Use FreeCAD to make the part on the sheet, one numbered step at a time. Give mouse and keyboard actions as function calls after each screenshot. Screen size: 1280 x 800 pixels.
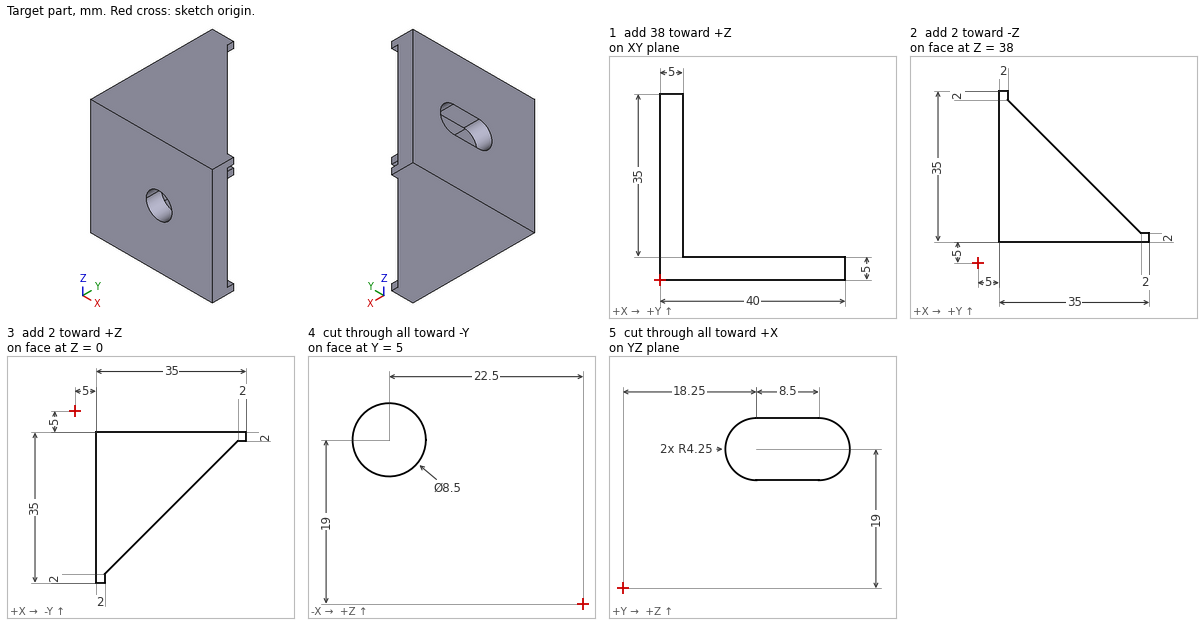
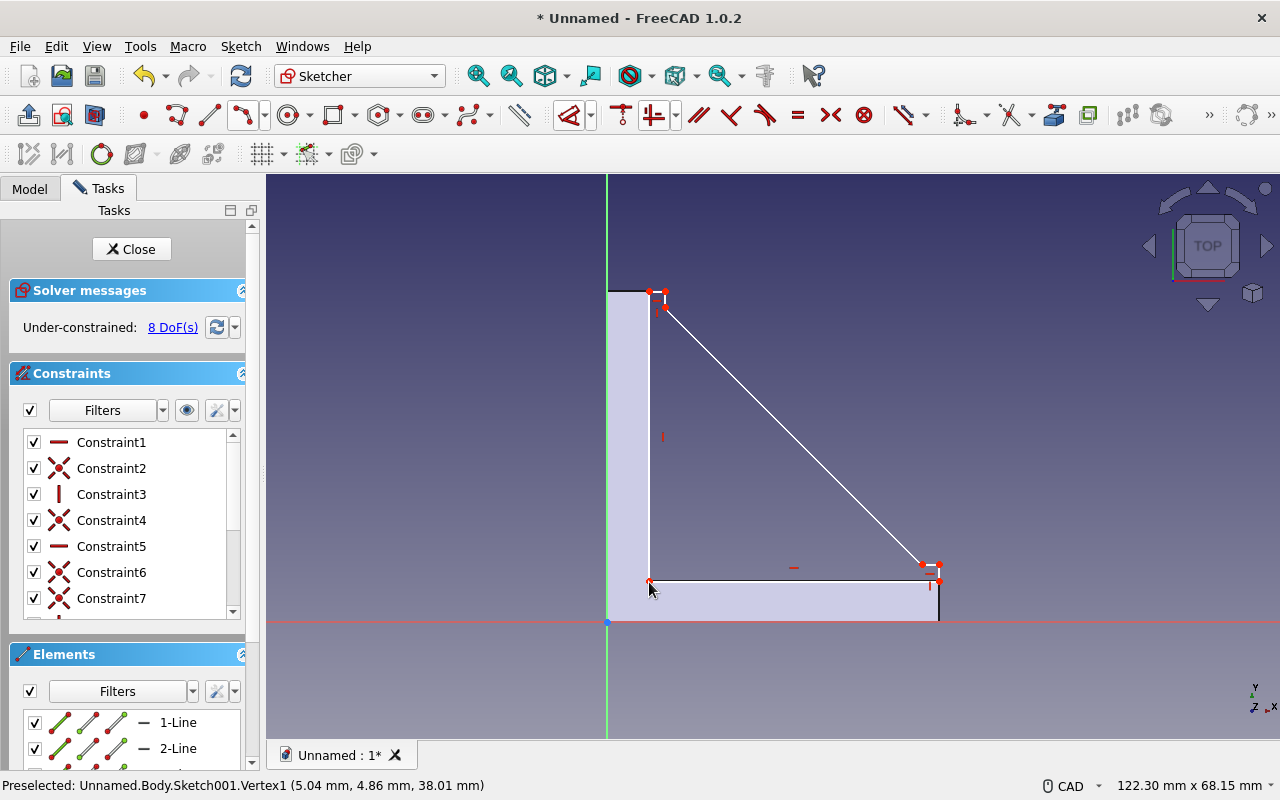
scroll(939, 574, up, 5)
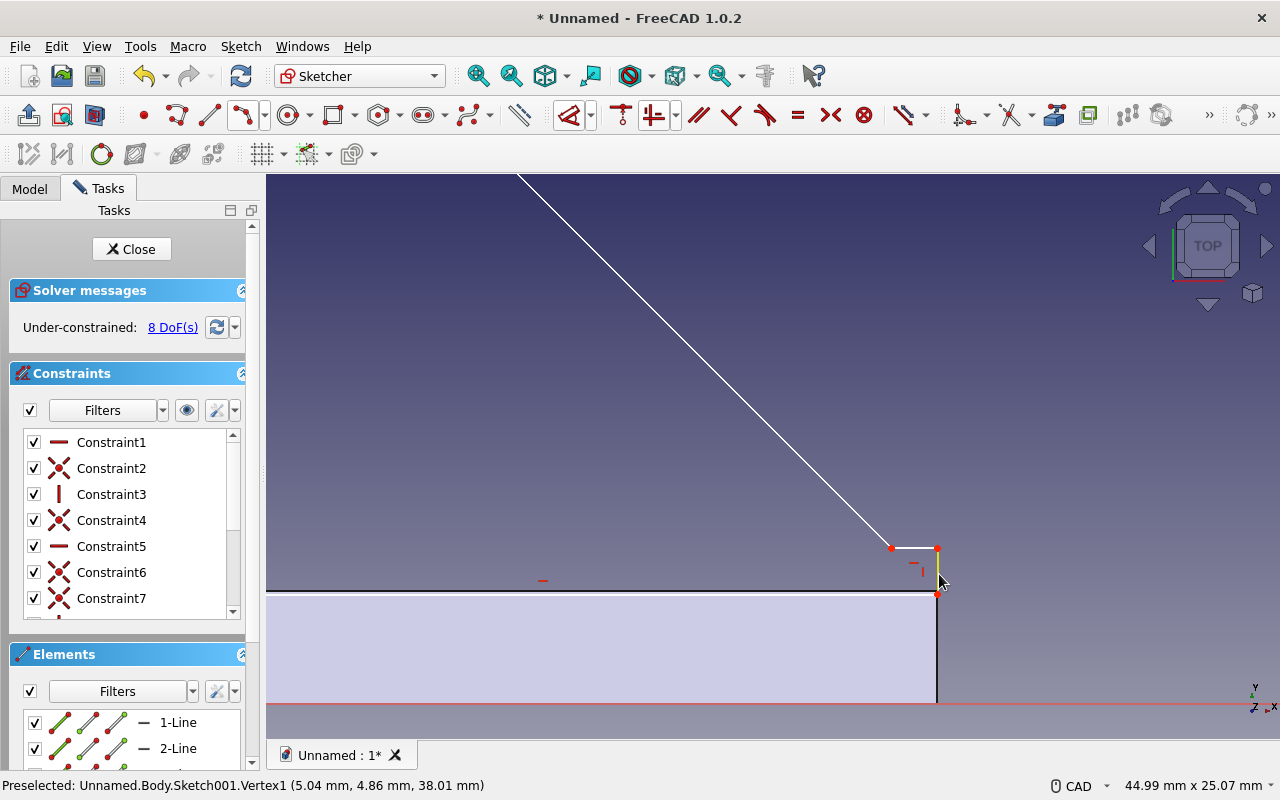
click(938, 571)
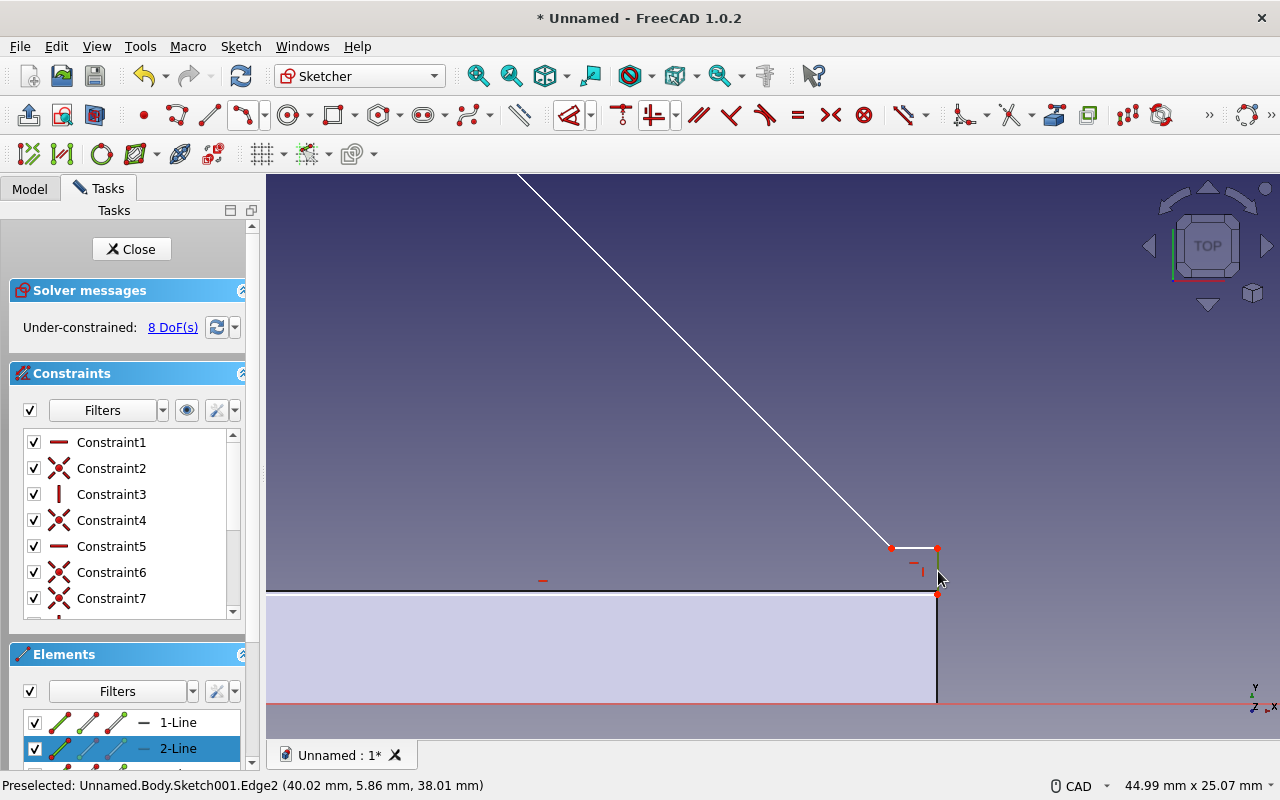
key(i)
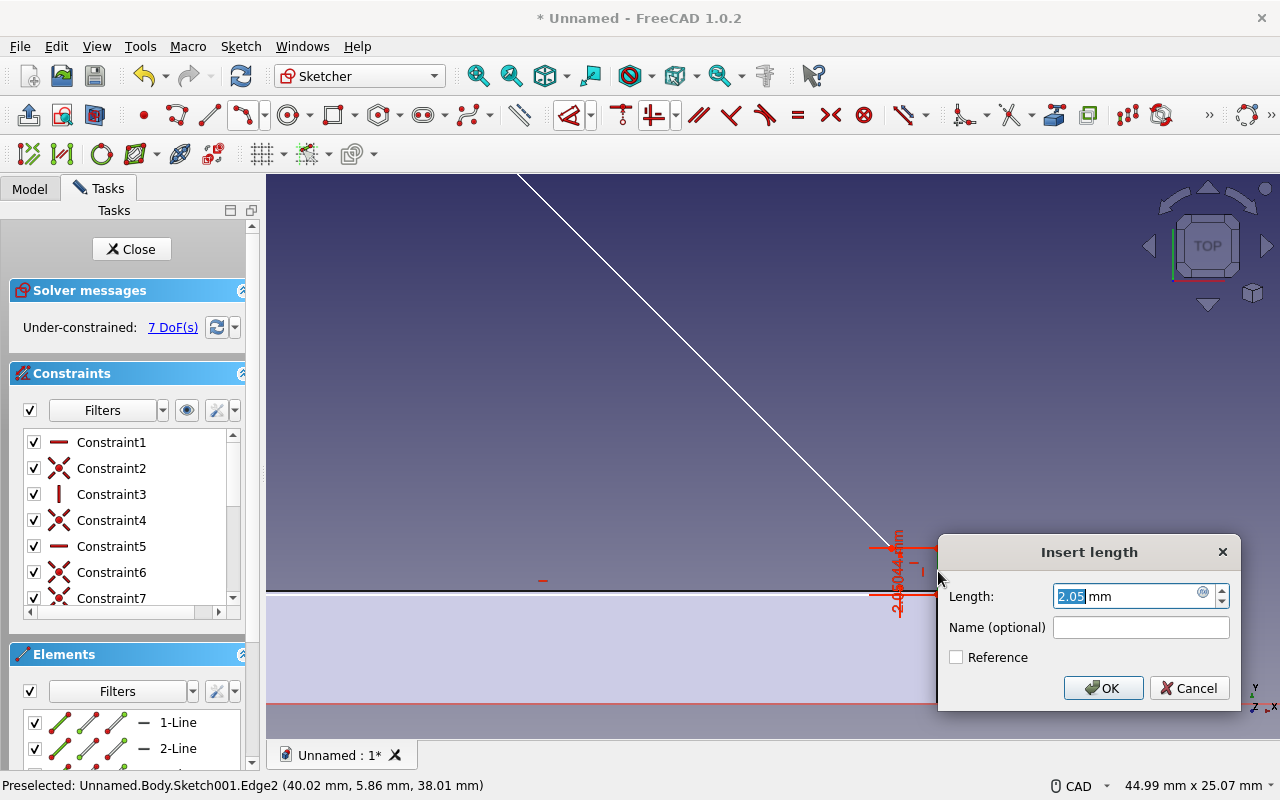
text(2)
key(Return)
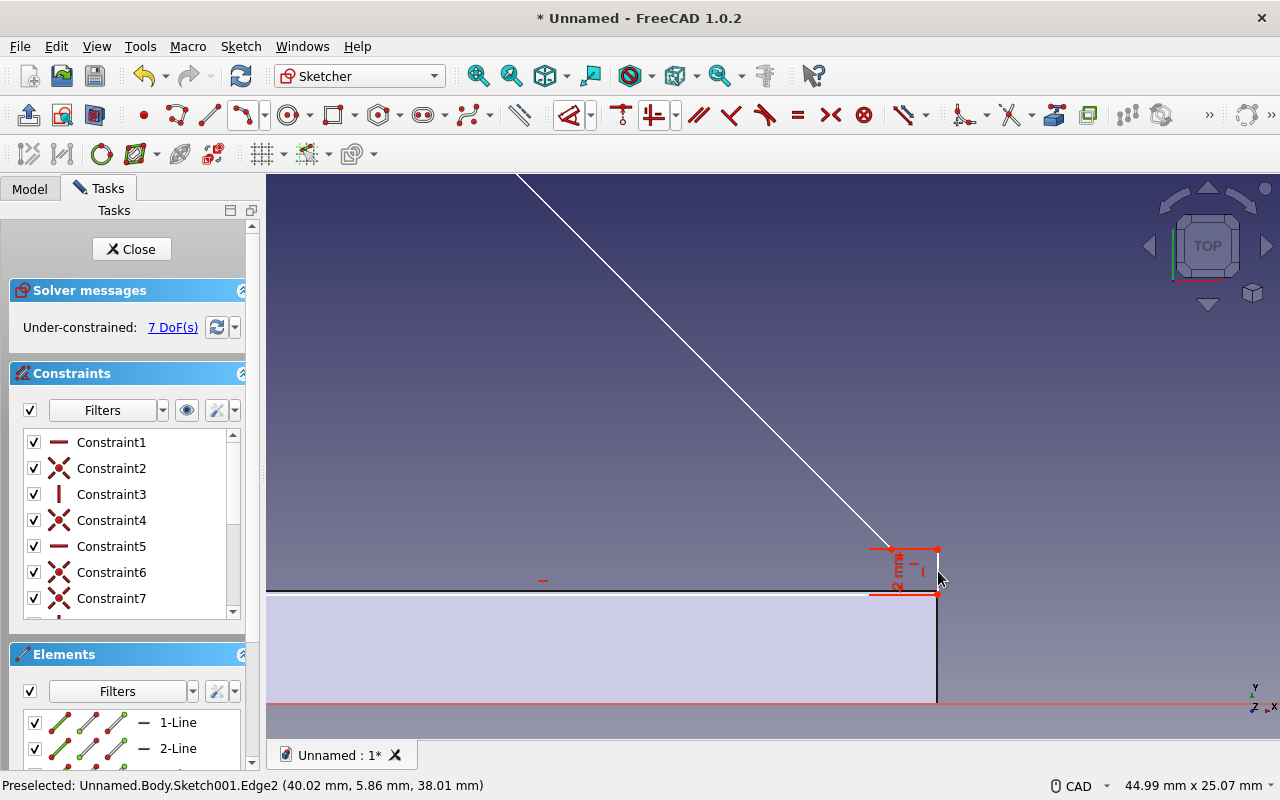
click(924, 549)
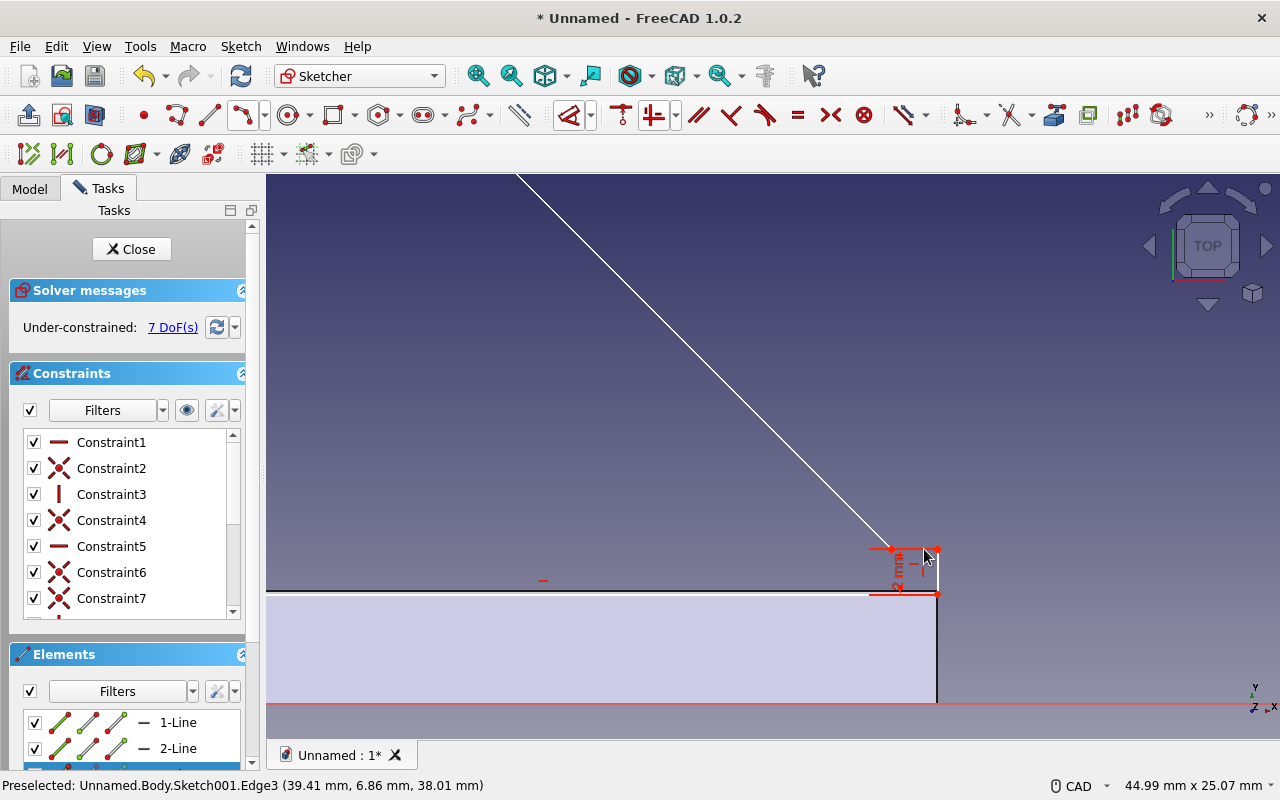
key(l)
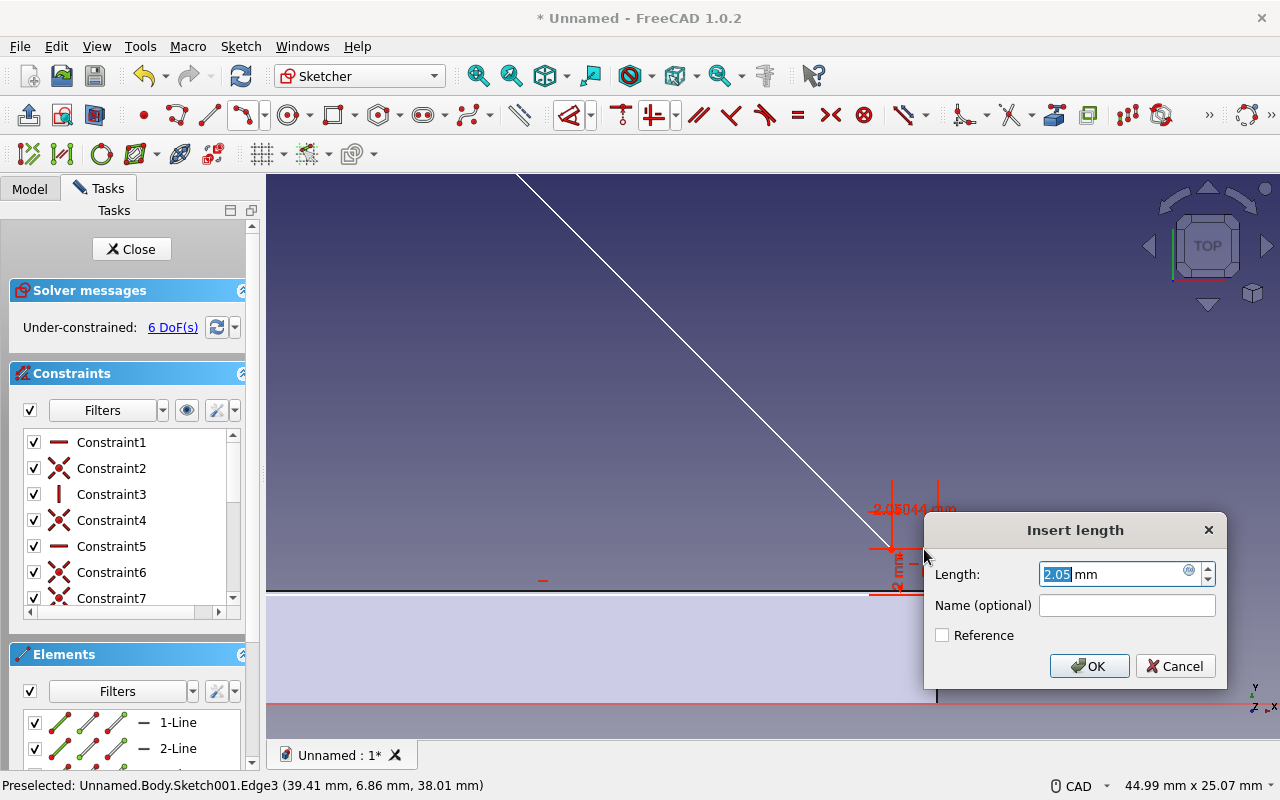
text(2)
key(Return)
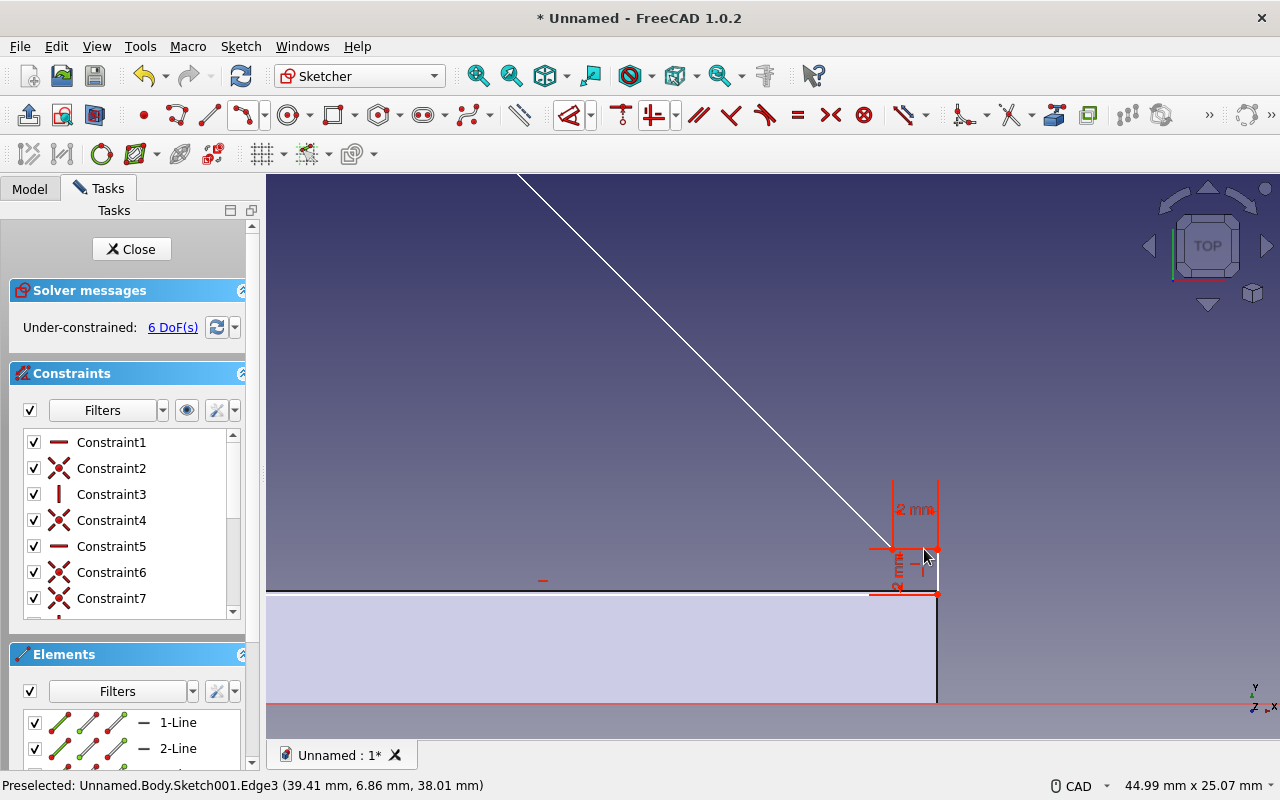
scroll(831, 575, down, 5)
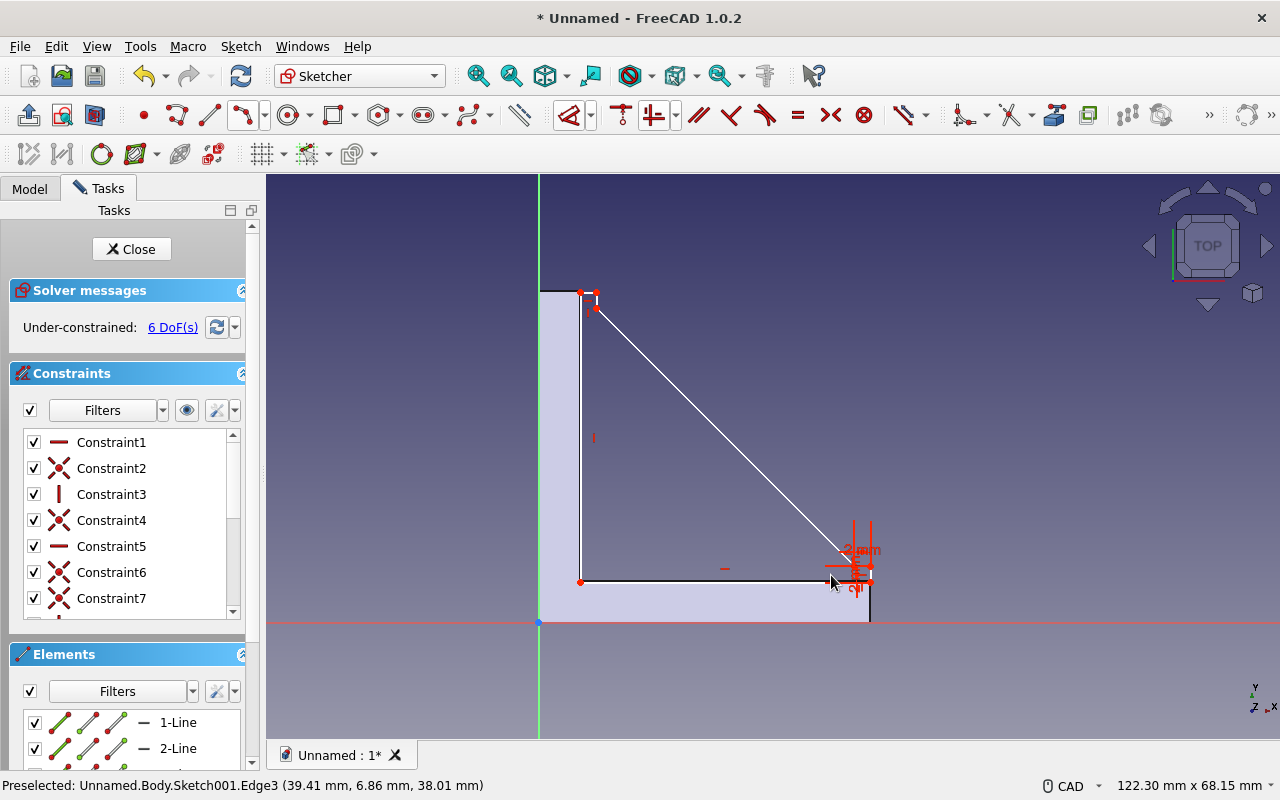
scroll(597, 304, up, 6)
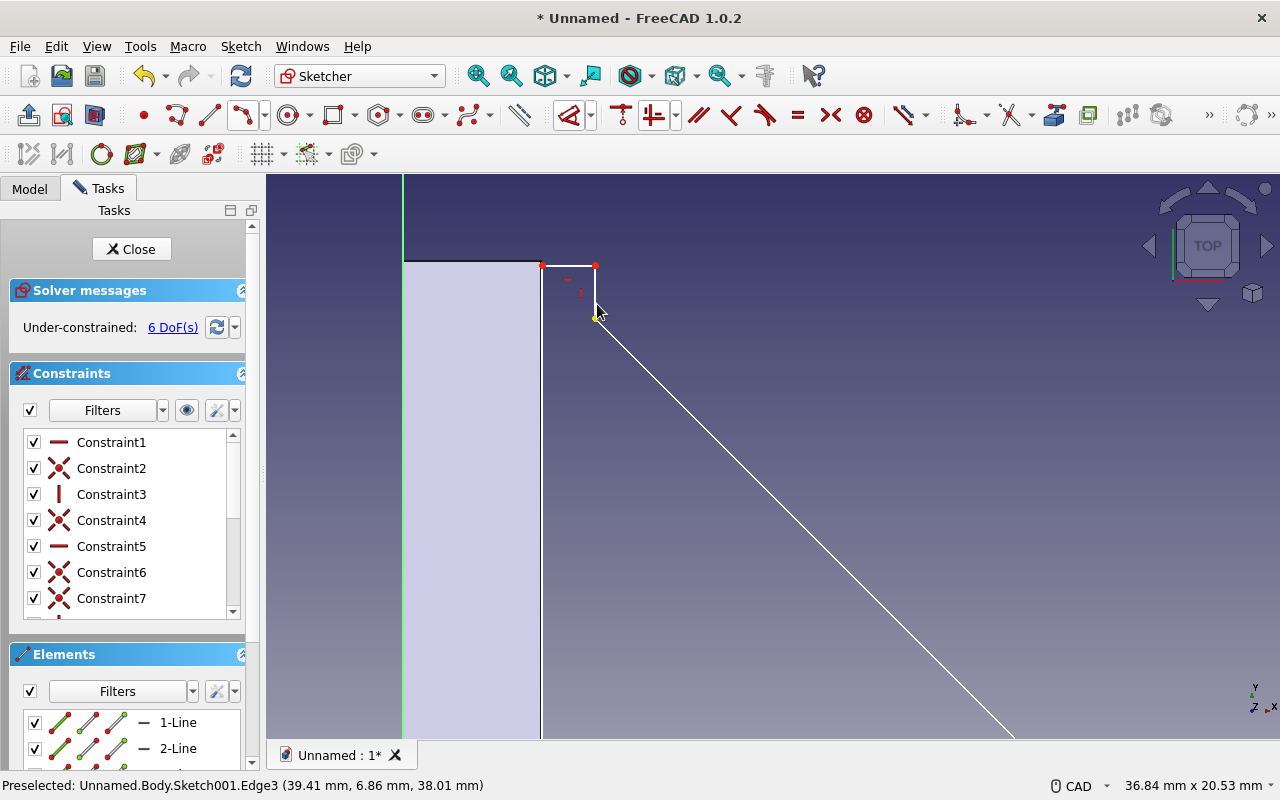
click(595, 303)